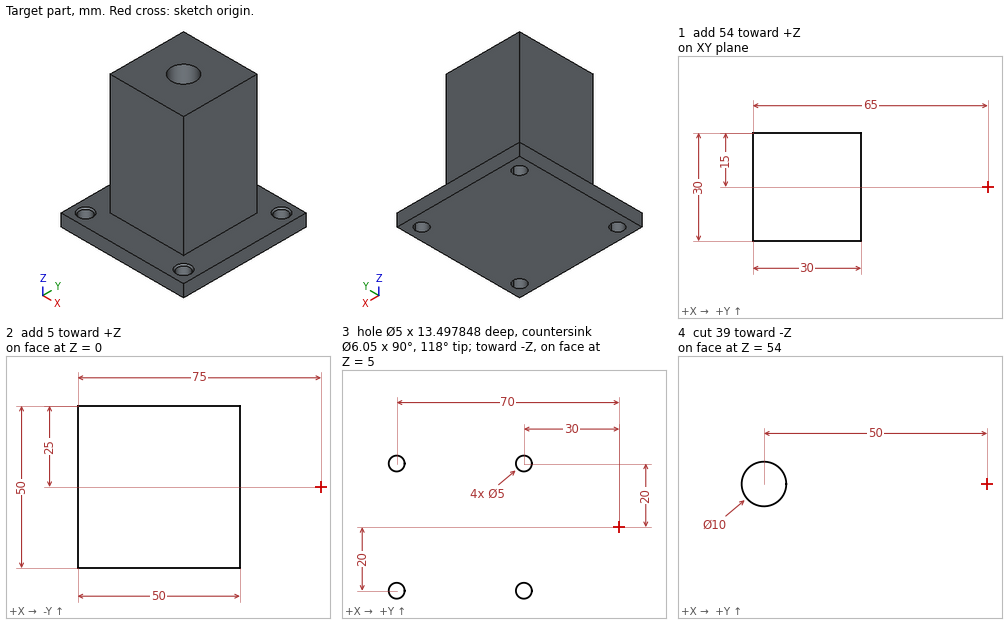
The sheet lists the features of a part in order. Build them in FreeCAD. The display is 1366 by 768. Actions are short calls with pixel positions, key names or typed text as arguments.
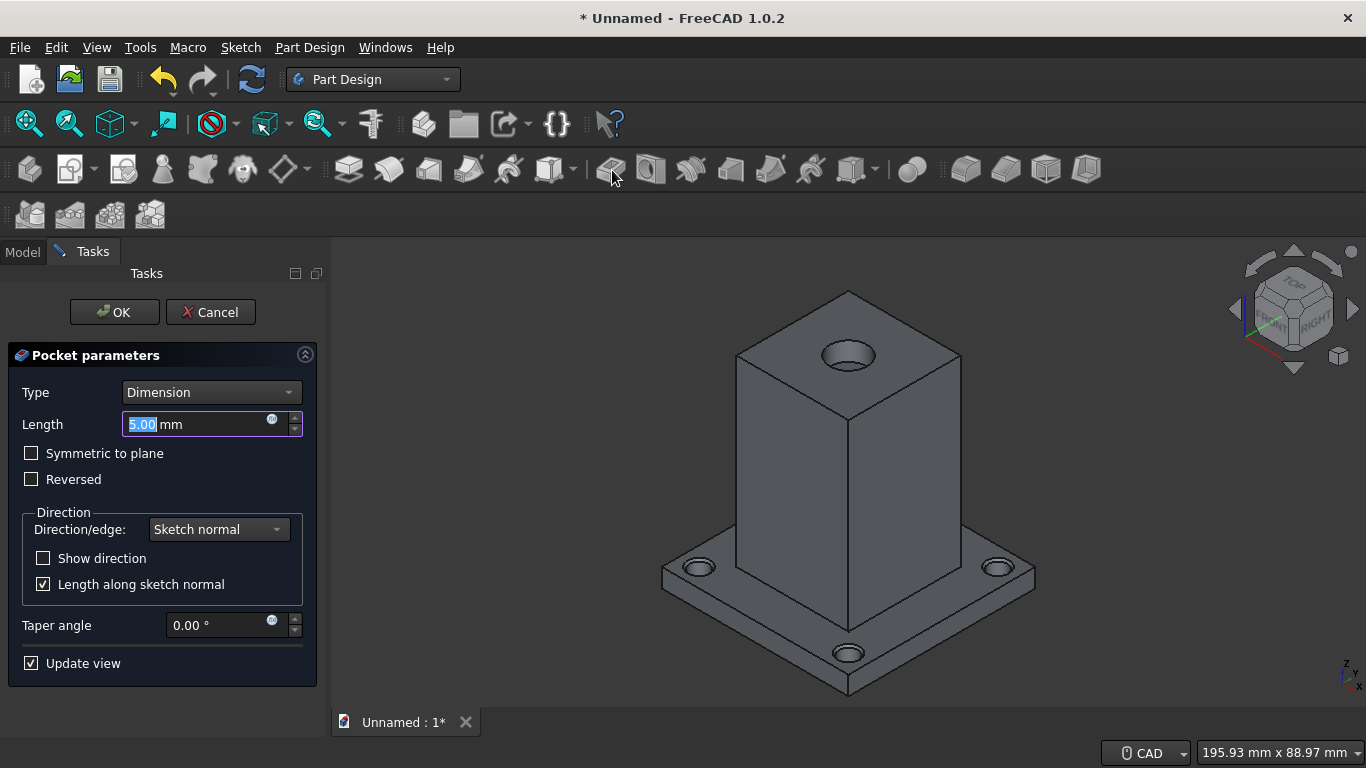
text(39)
key(Tab)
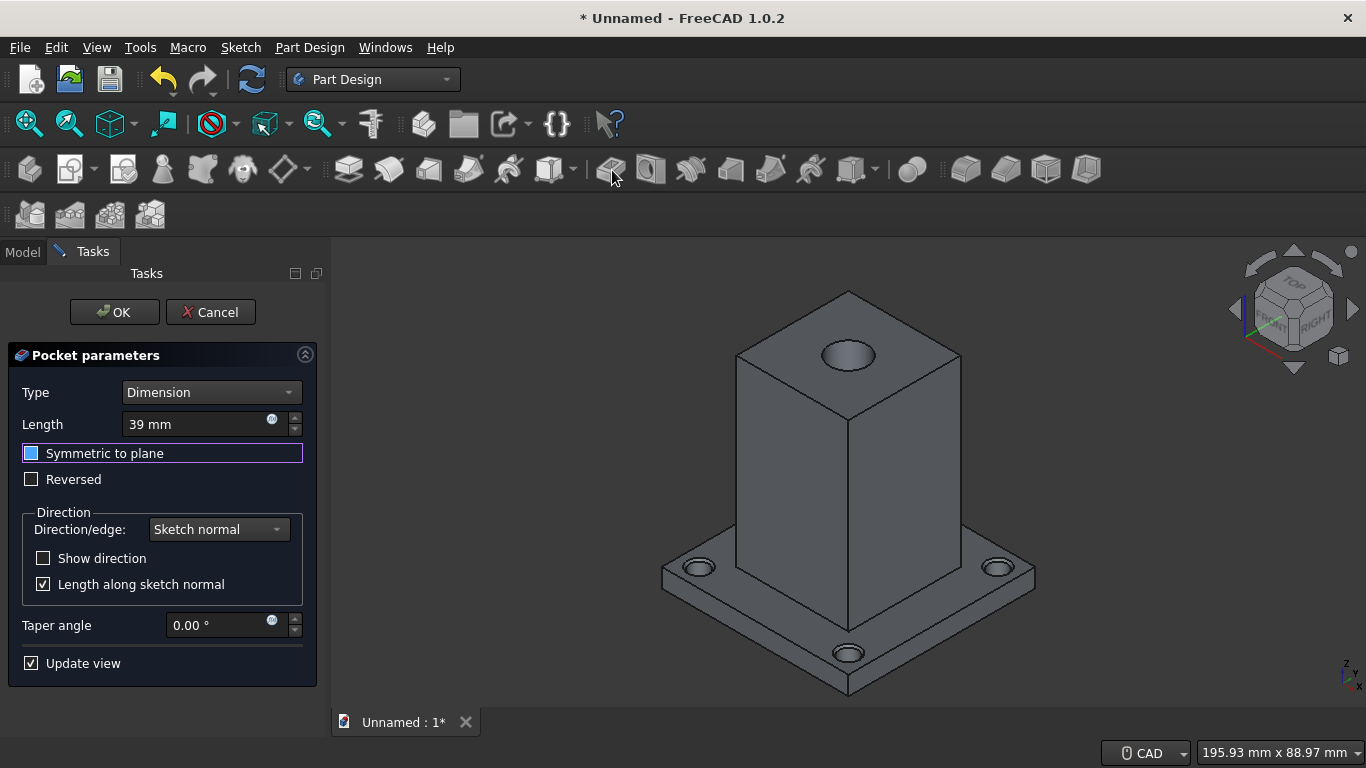
click(115, 312)